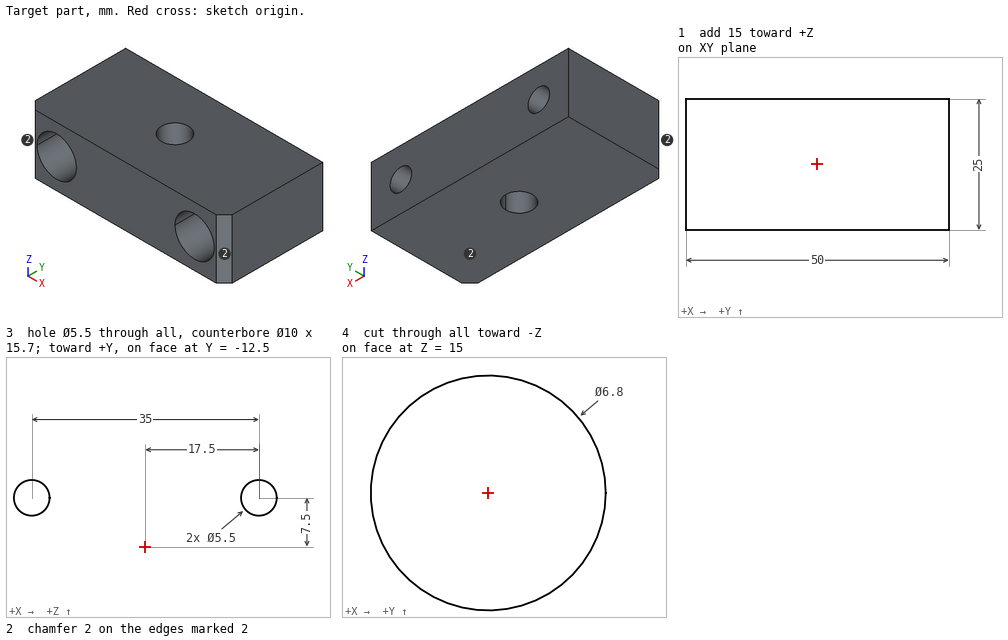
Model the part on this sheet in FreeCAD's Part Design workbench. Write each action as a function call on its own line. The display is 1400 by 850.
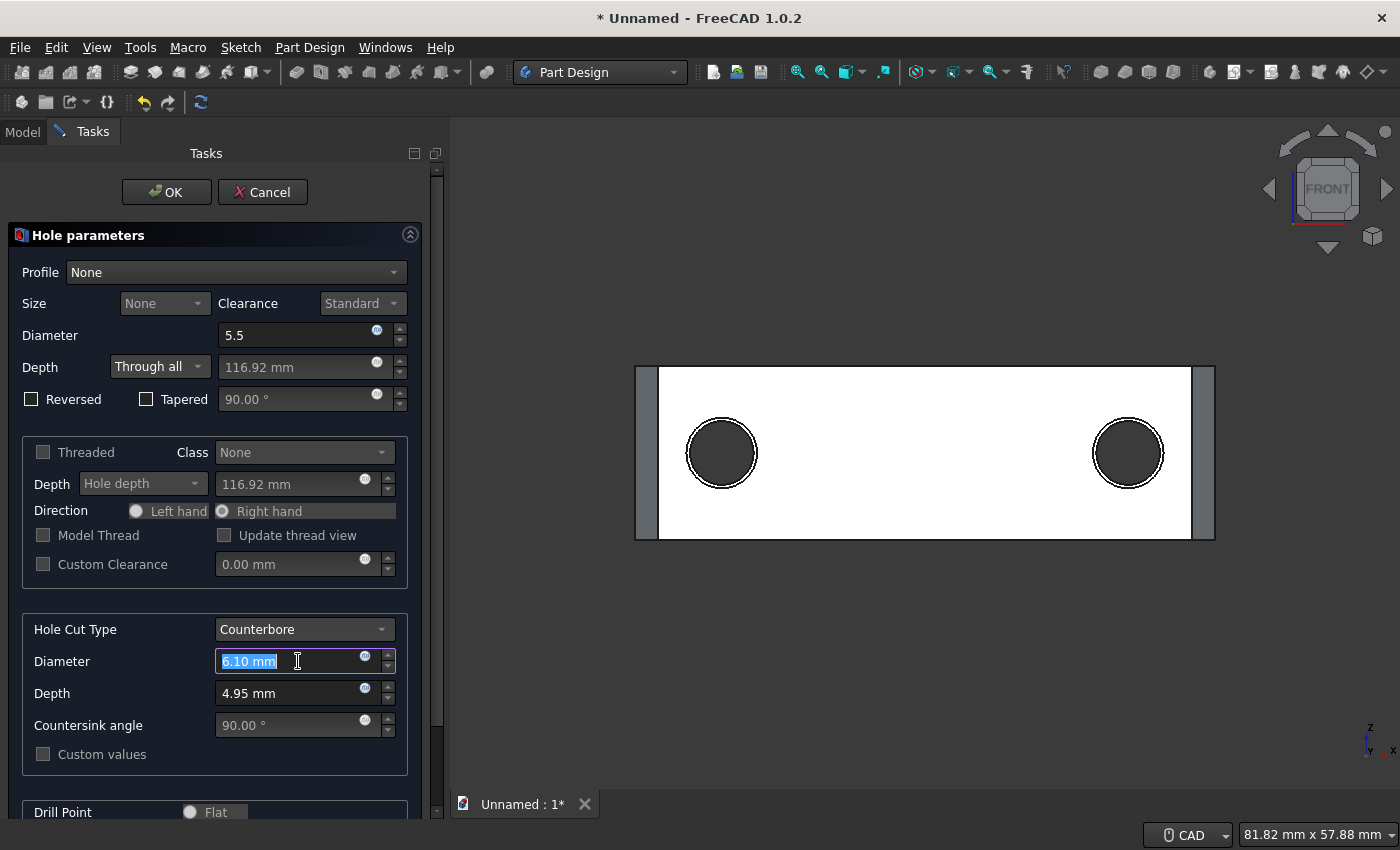
text(10)
key(Tab)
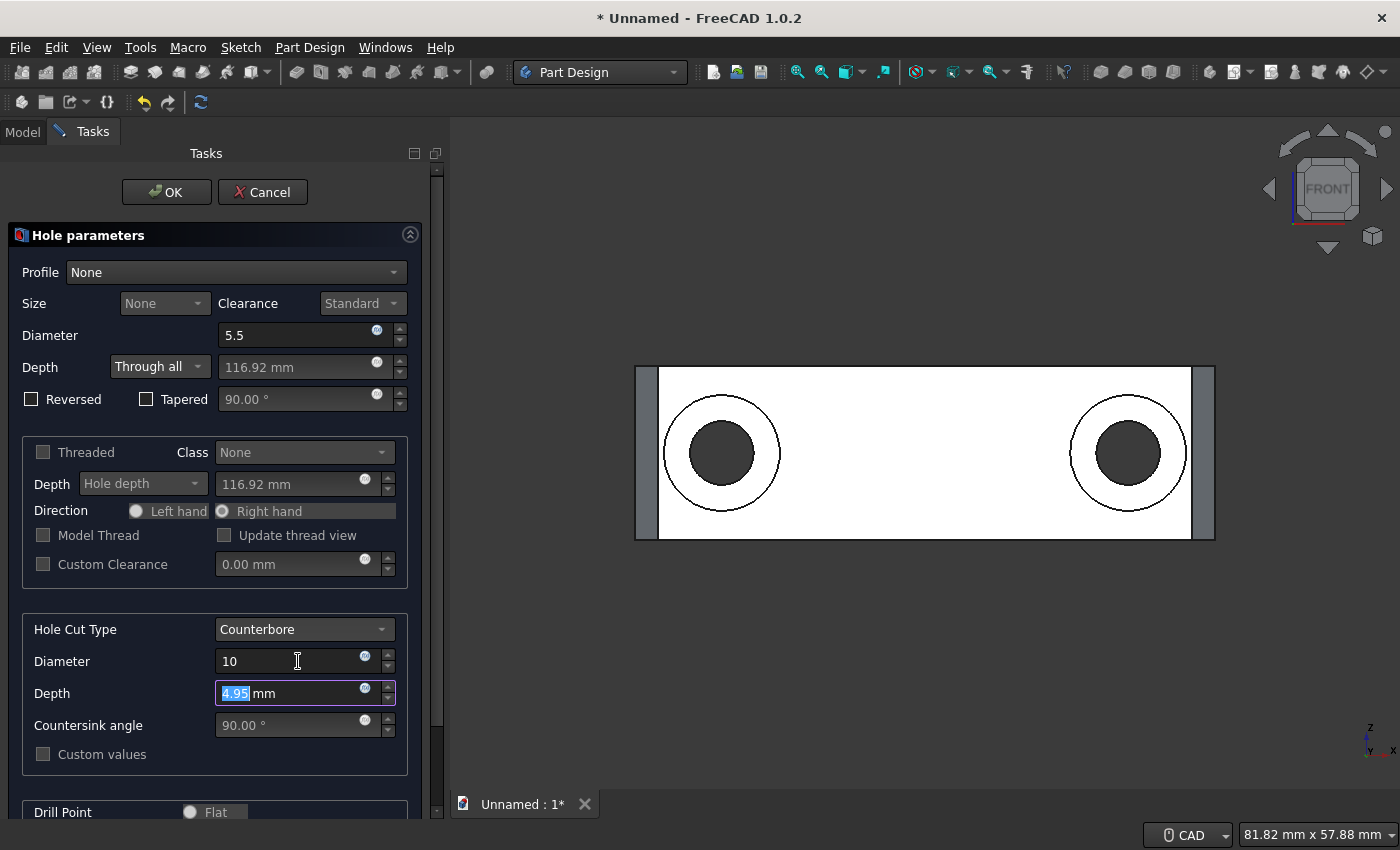
text(15.7)
key(Tab)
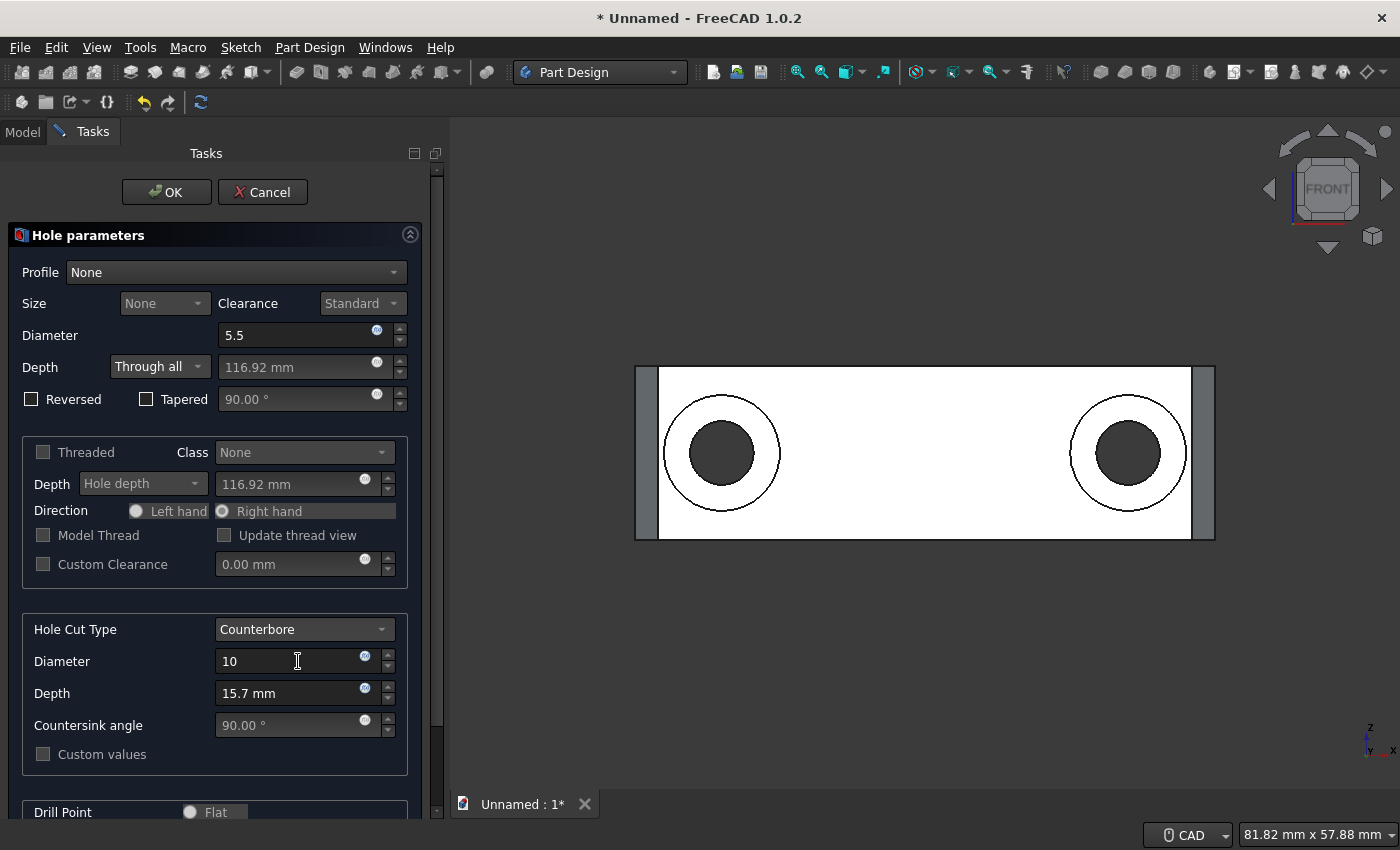
click(167, 192)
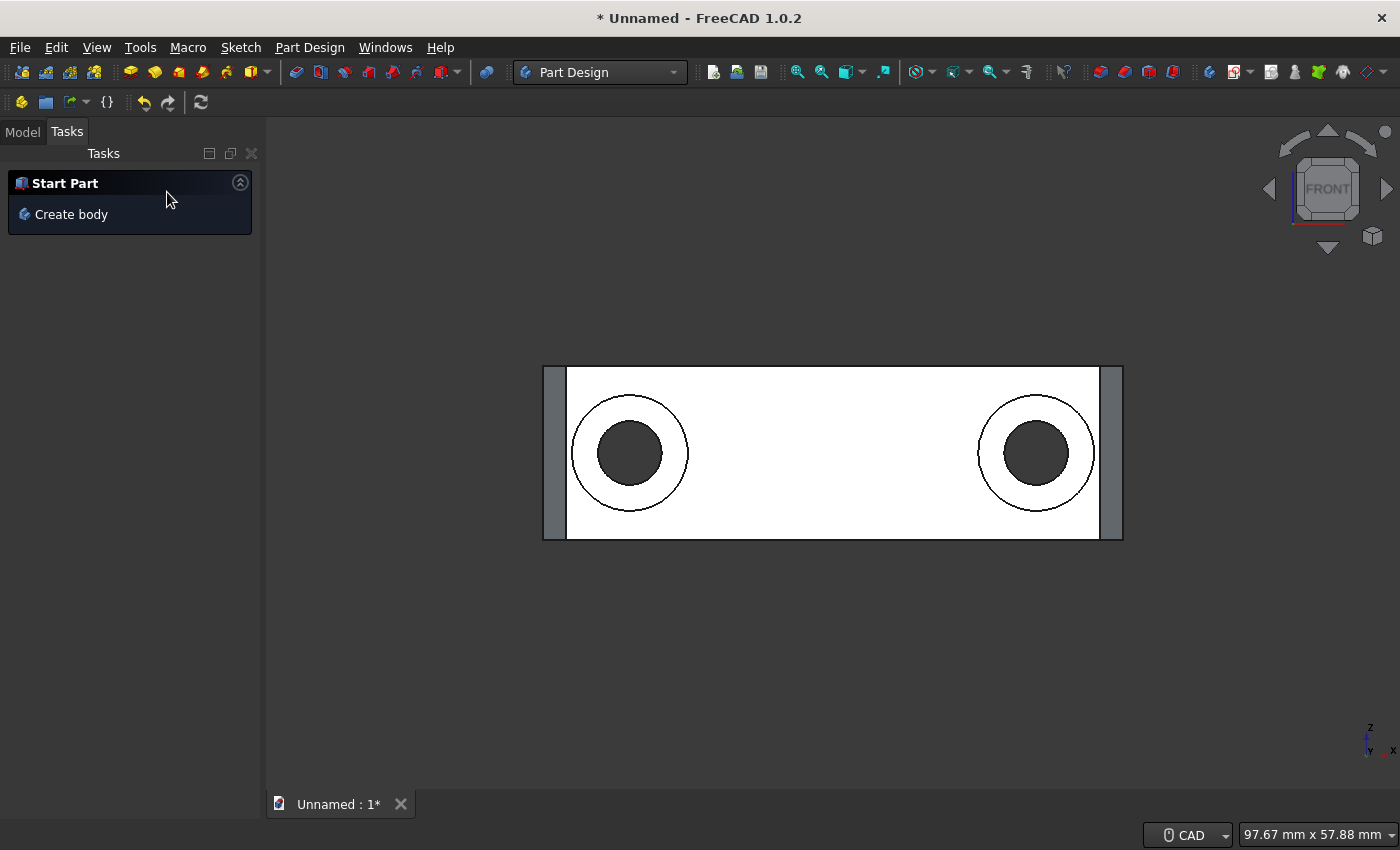
key(0)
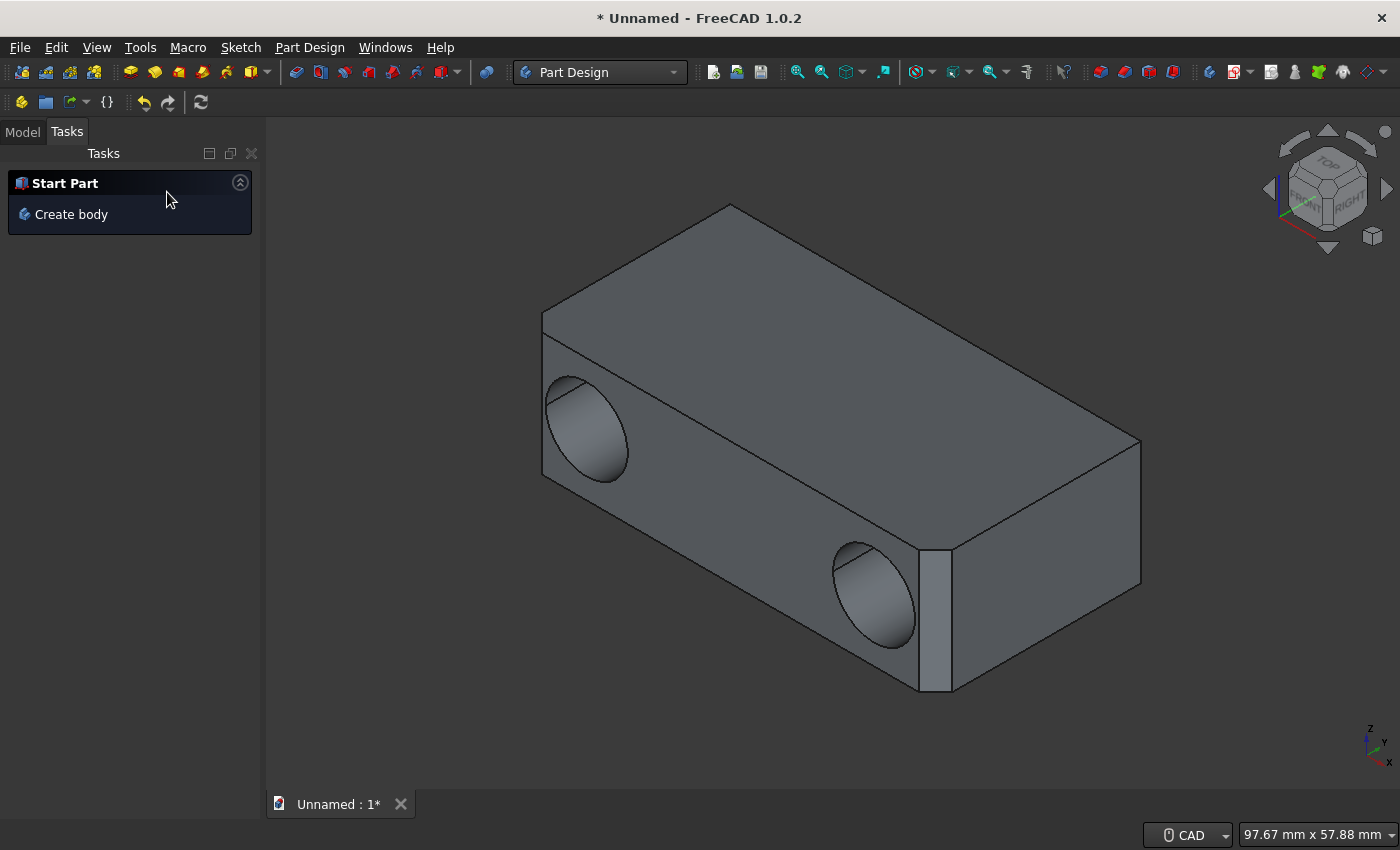
click(892, 415)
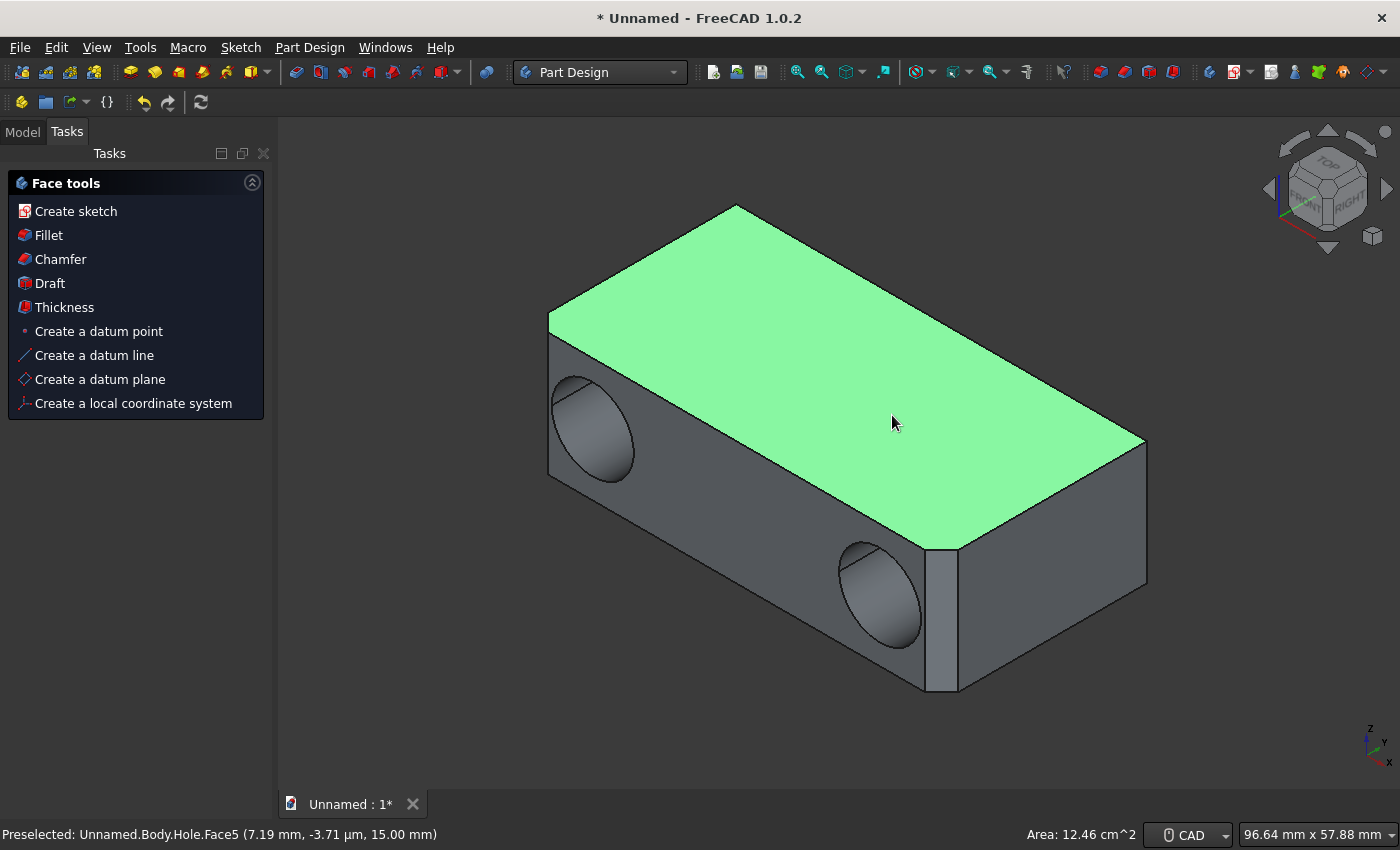
click(1234, 72)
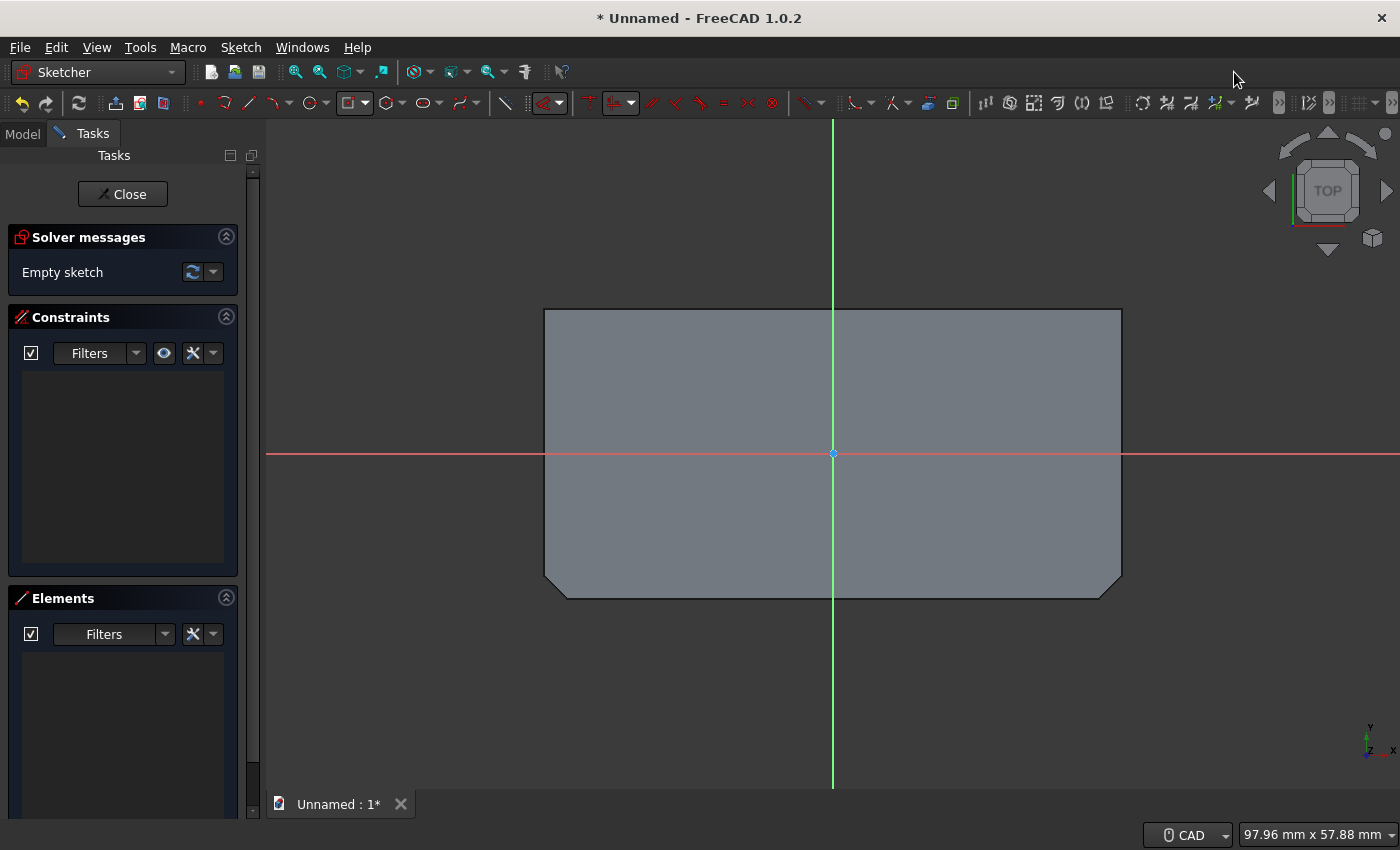
scroll(847, 454, up, 9)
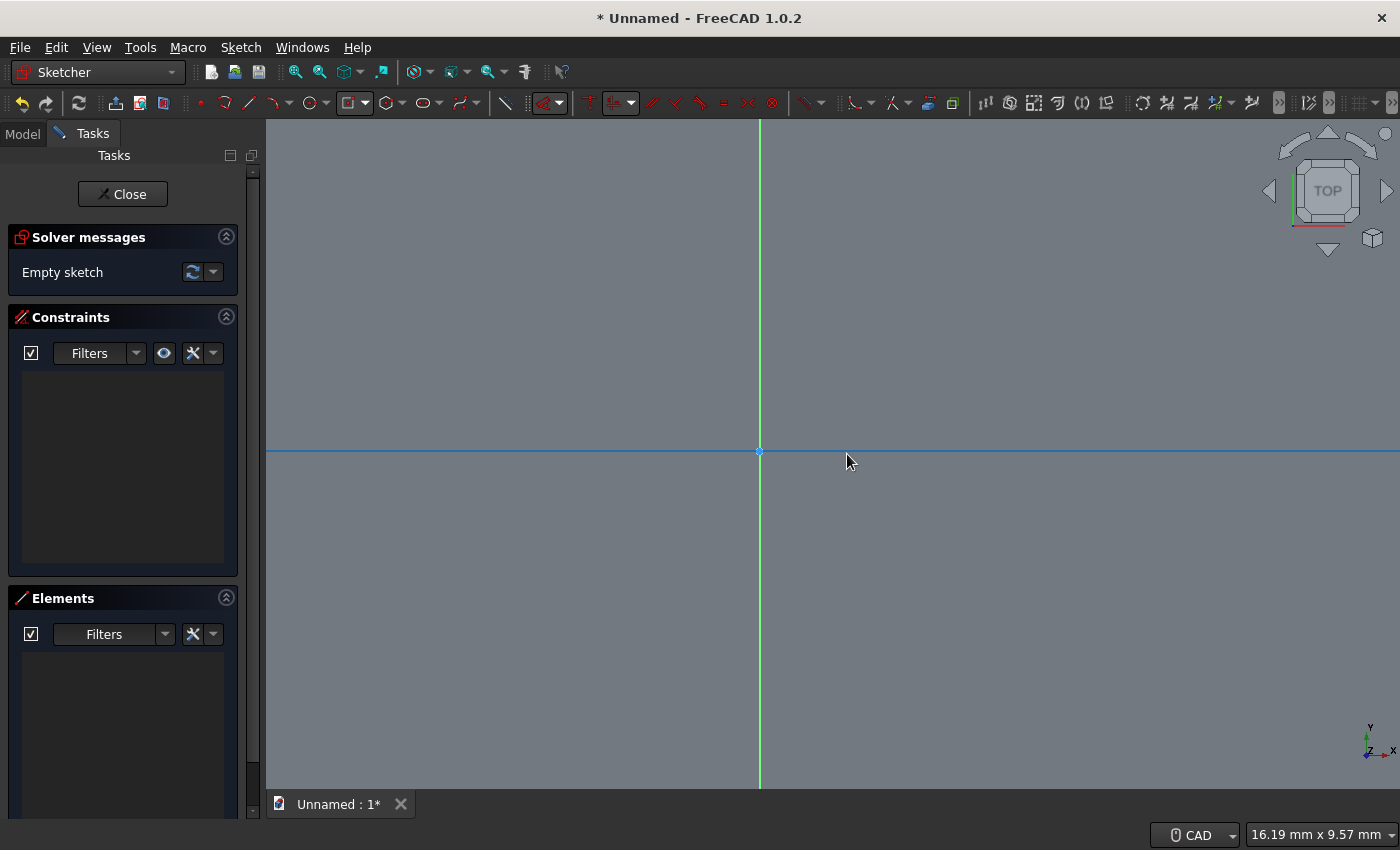
key(g)
key(c)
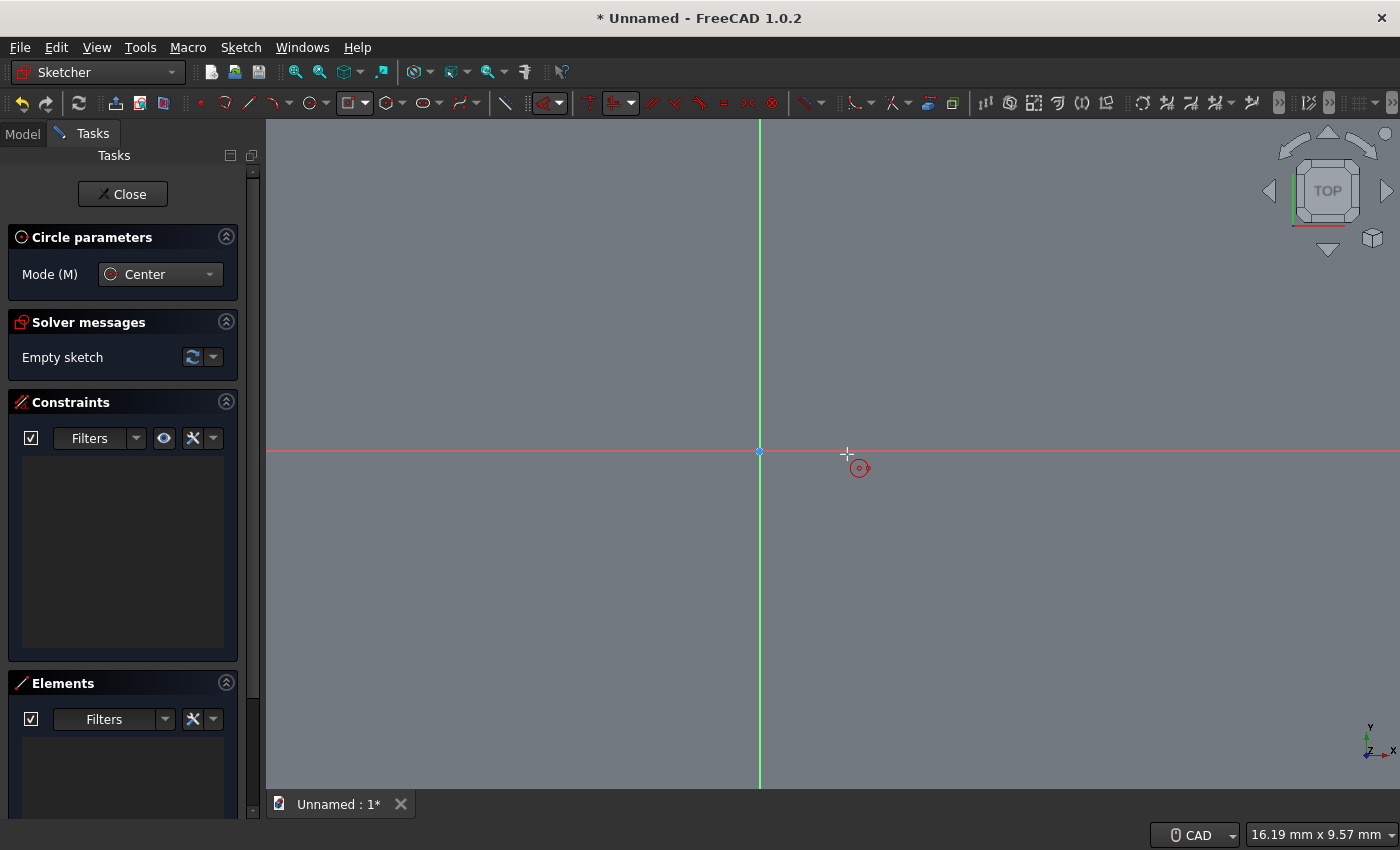
click(760, 451)
move(928, 283)